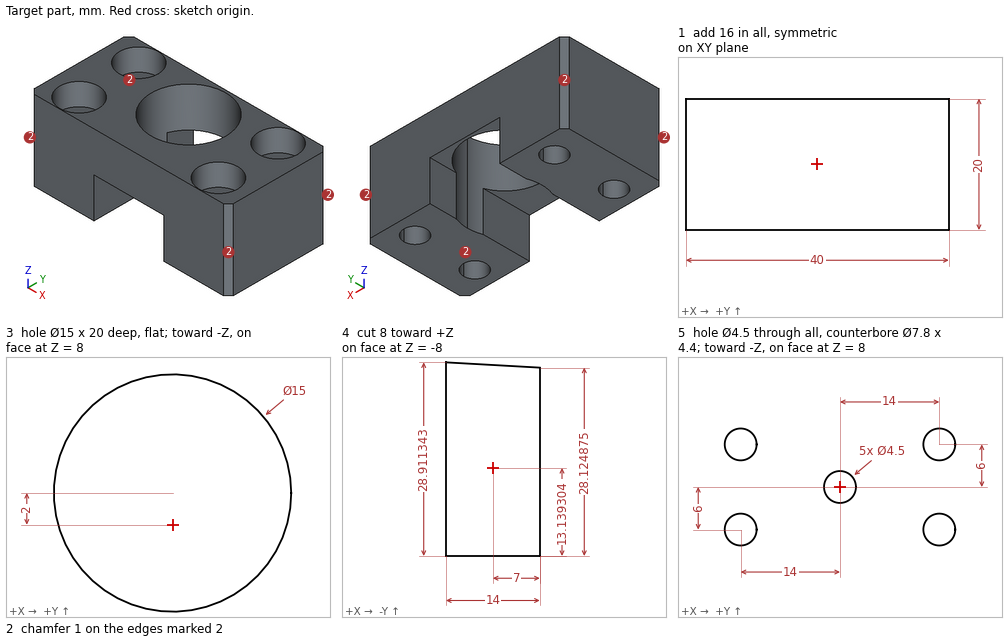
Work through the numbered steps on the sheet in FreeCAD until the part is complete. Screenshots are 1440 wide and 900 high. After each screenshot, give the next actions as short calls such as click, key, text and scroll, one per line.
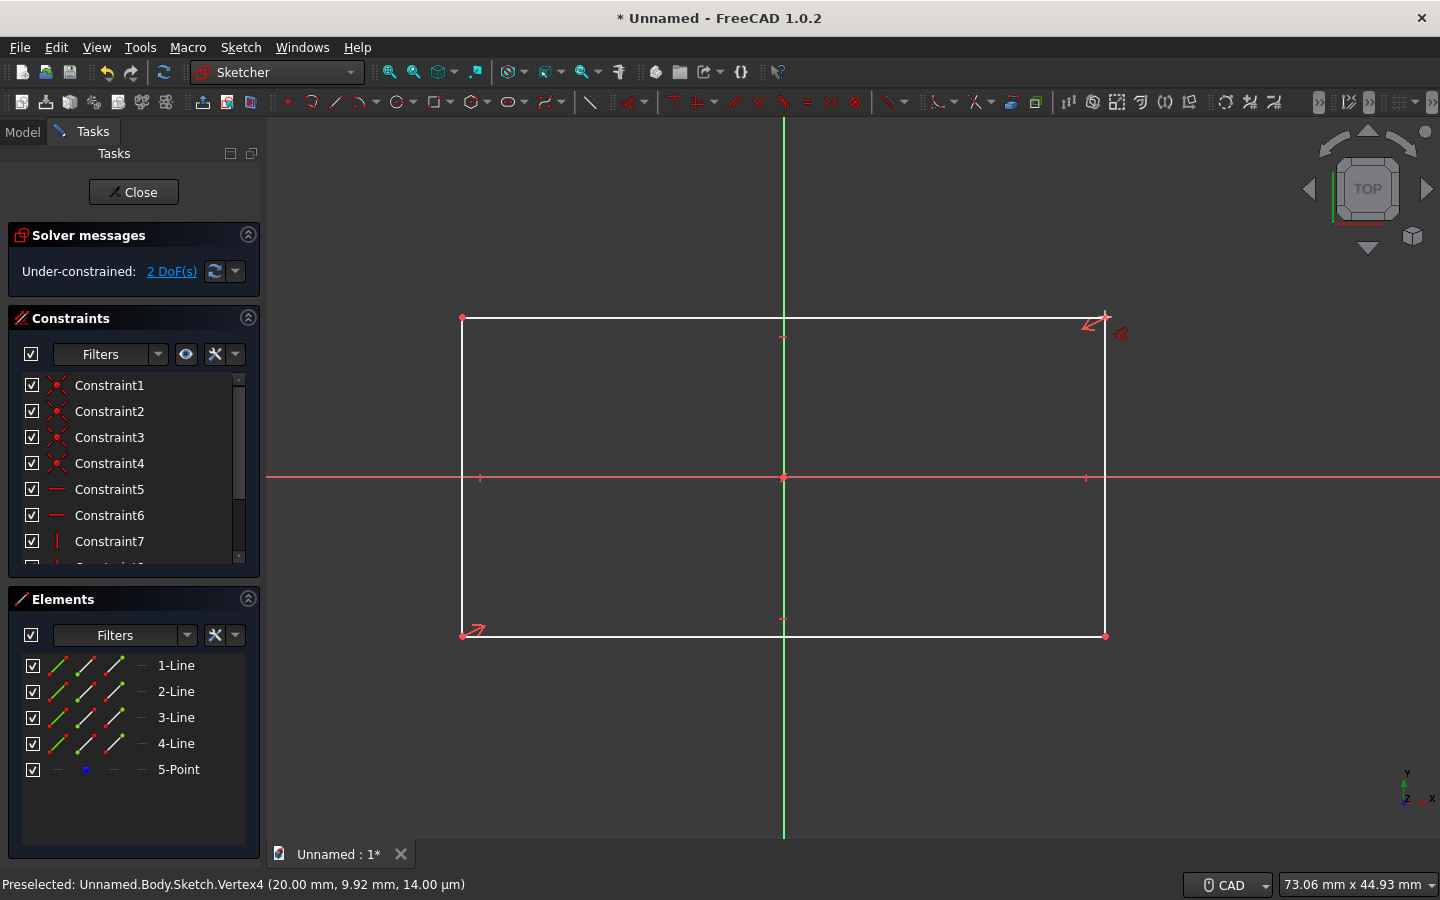
click(655, 637)
click(636, 671)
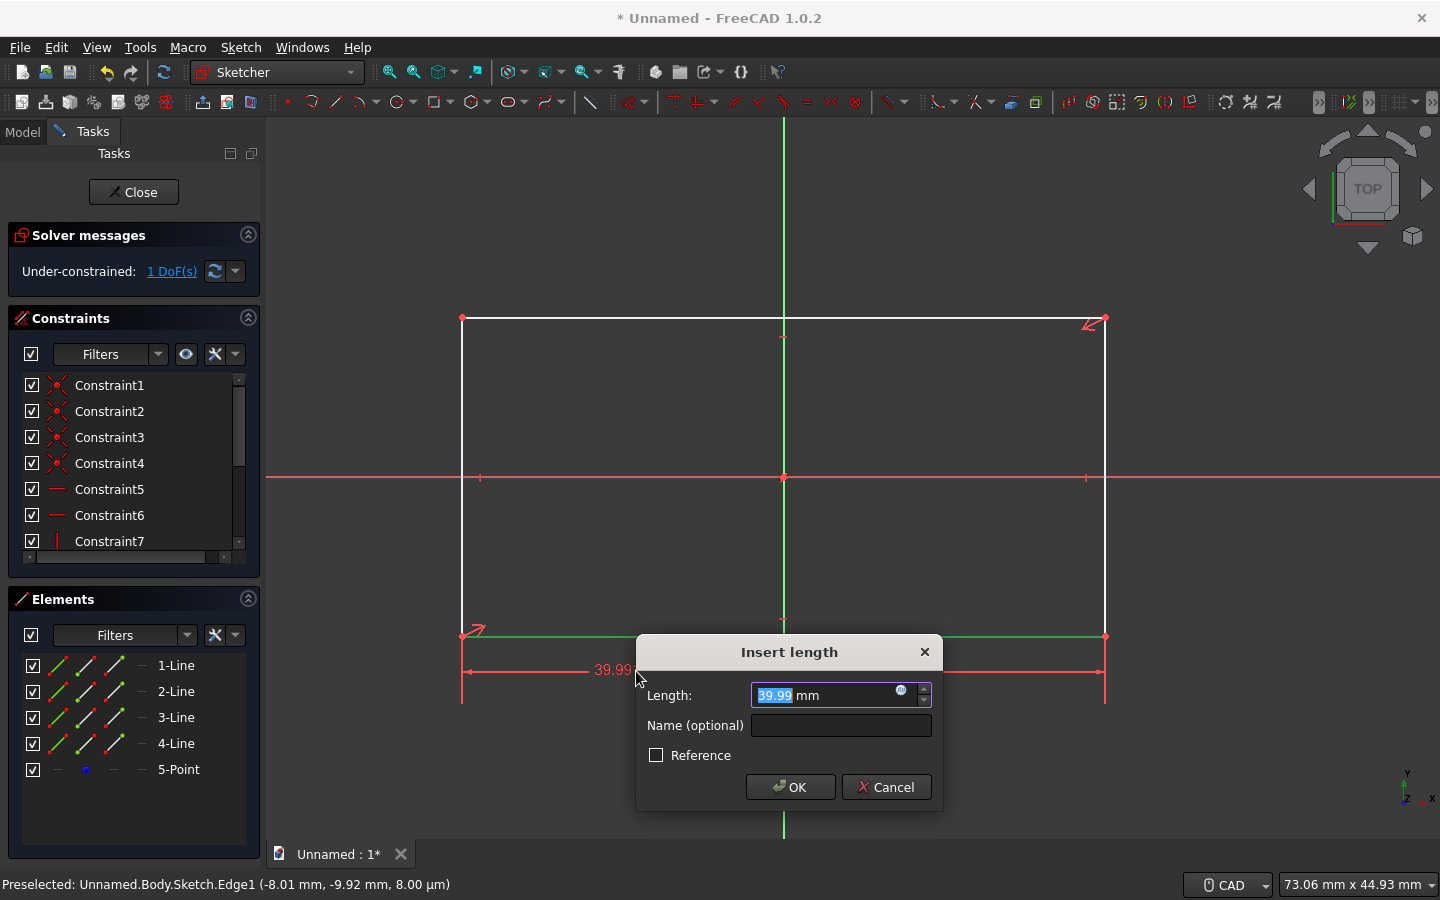
text(40)
key(Return)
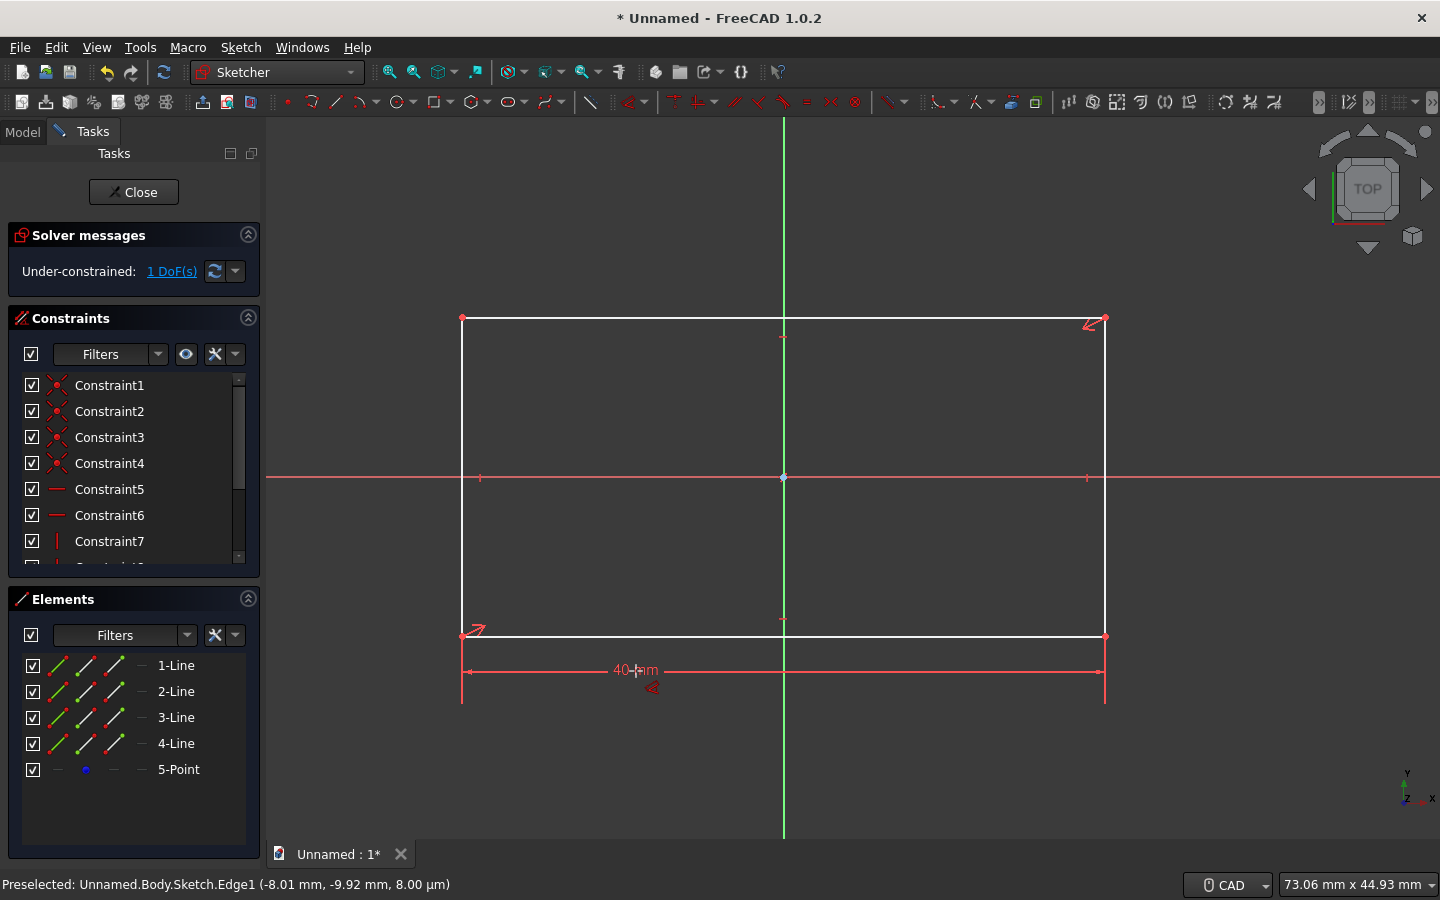
click(1105, 541)
click(1139, 404)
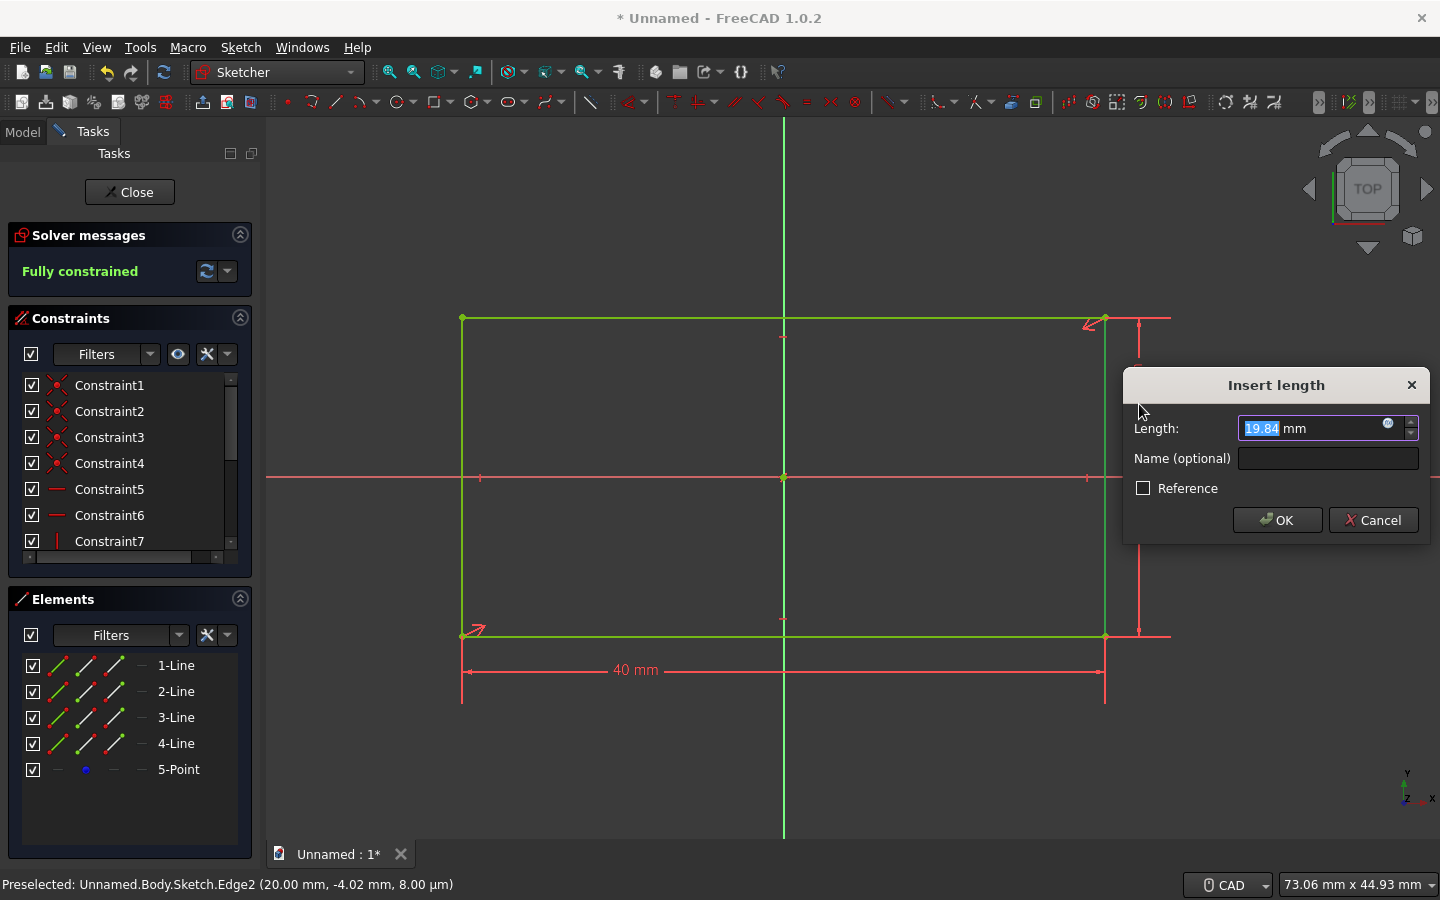
text(20)
key(Return)
key(Escape)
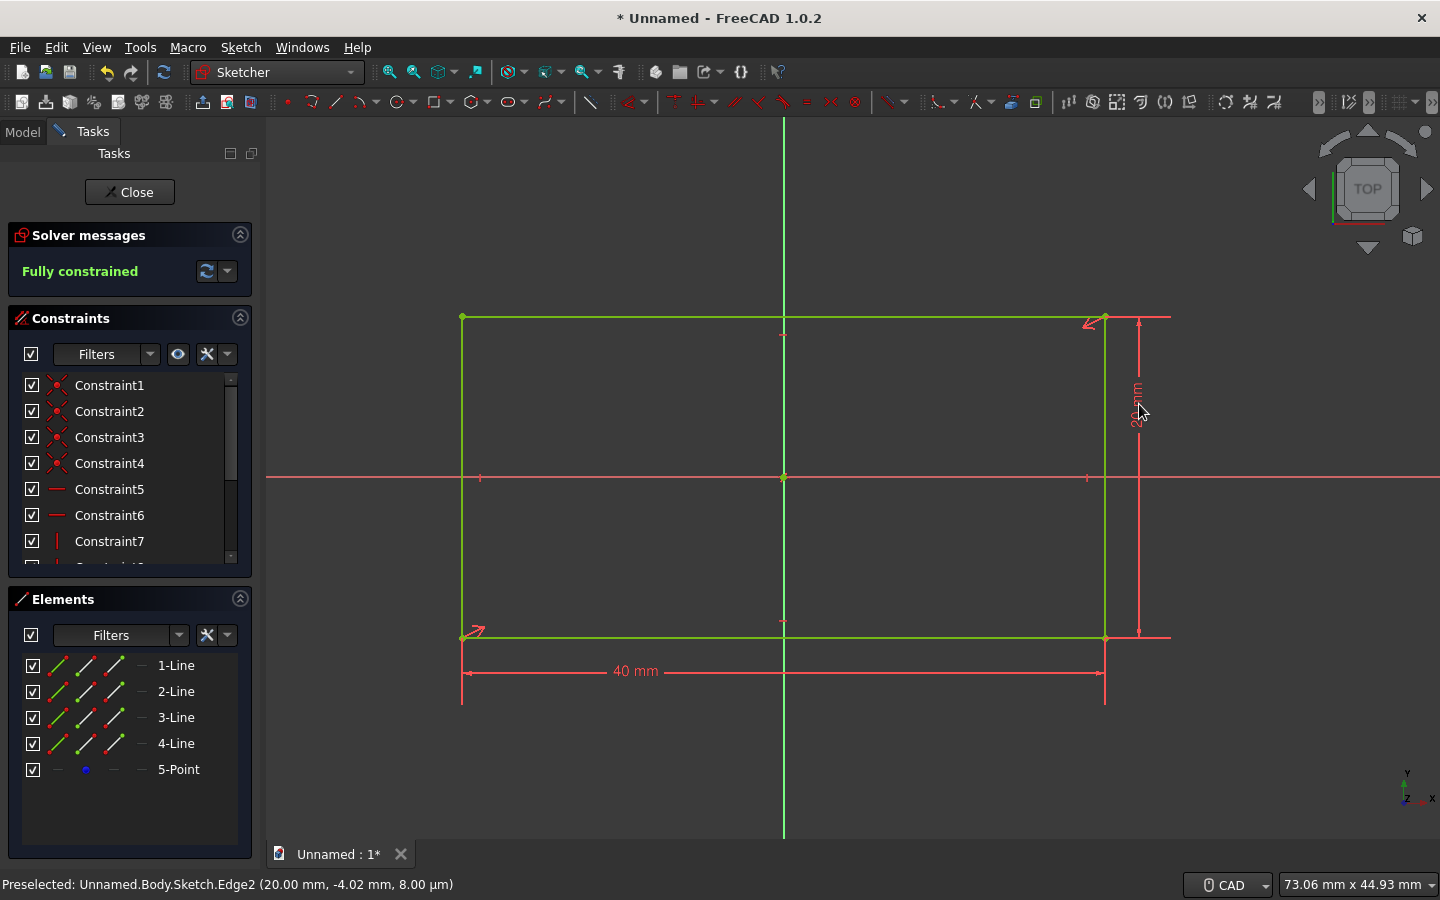
click(130, 192)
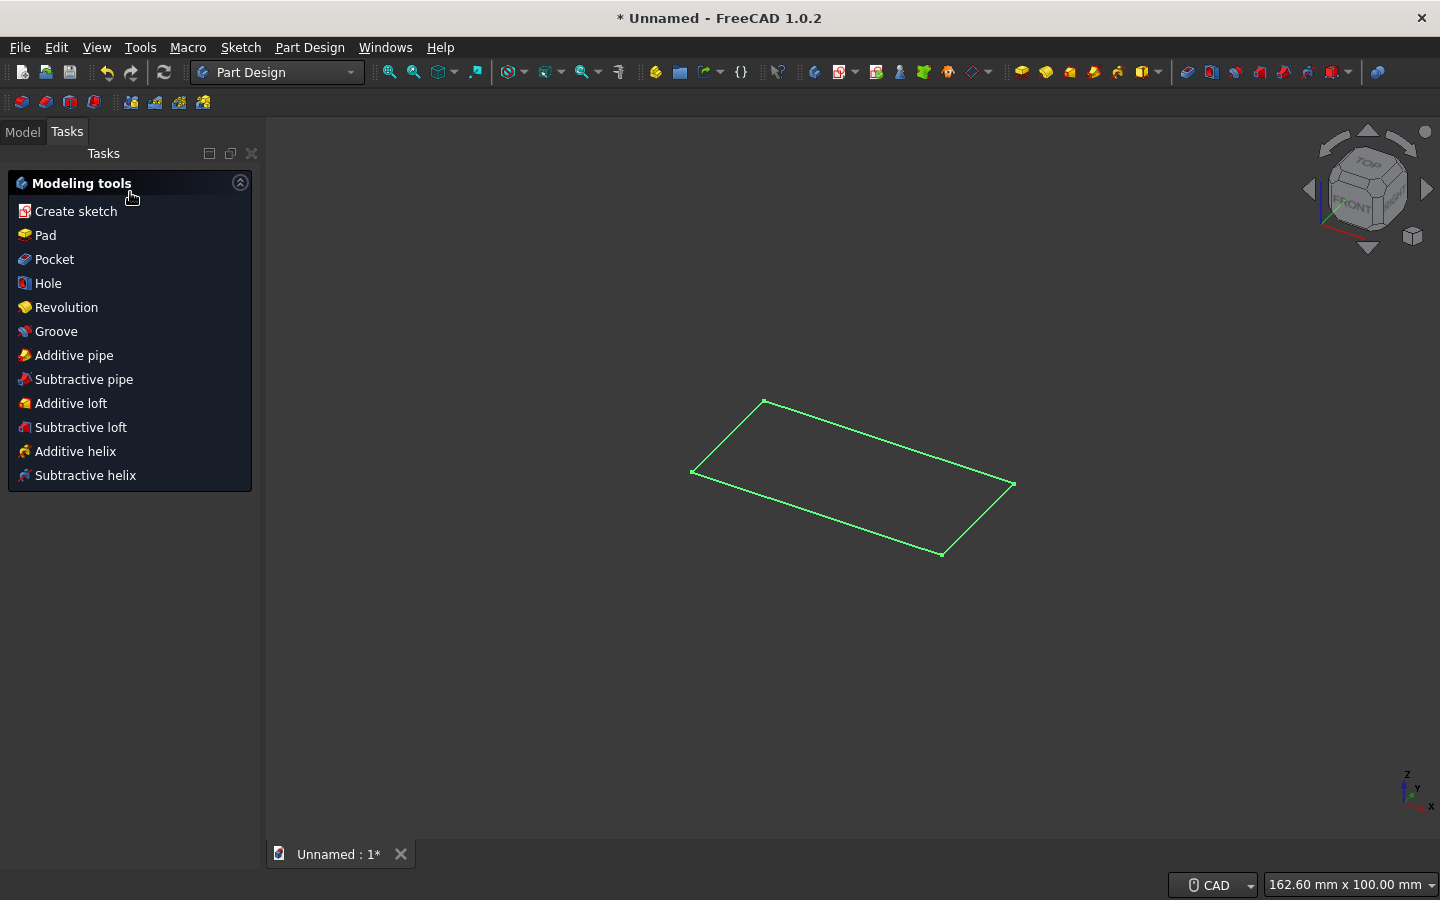
click(1022, 72)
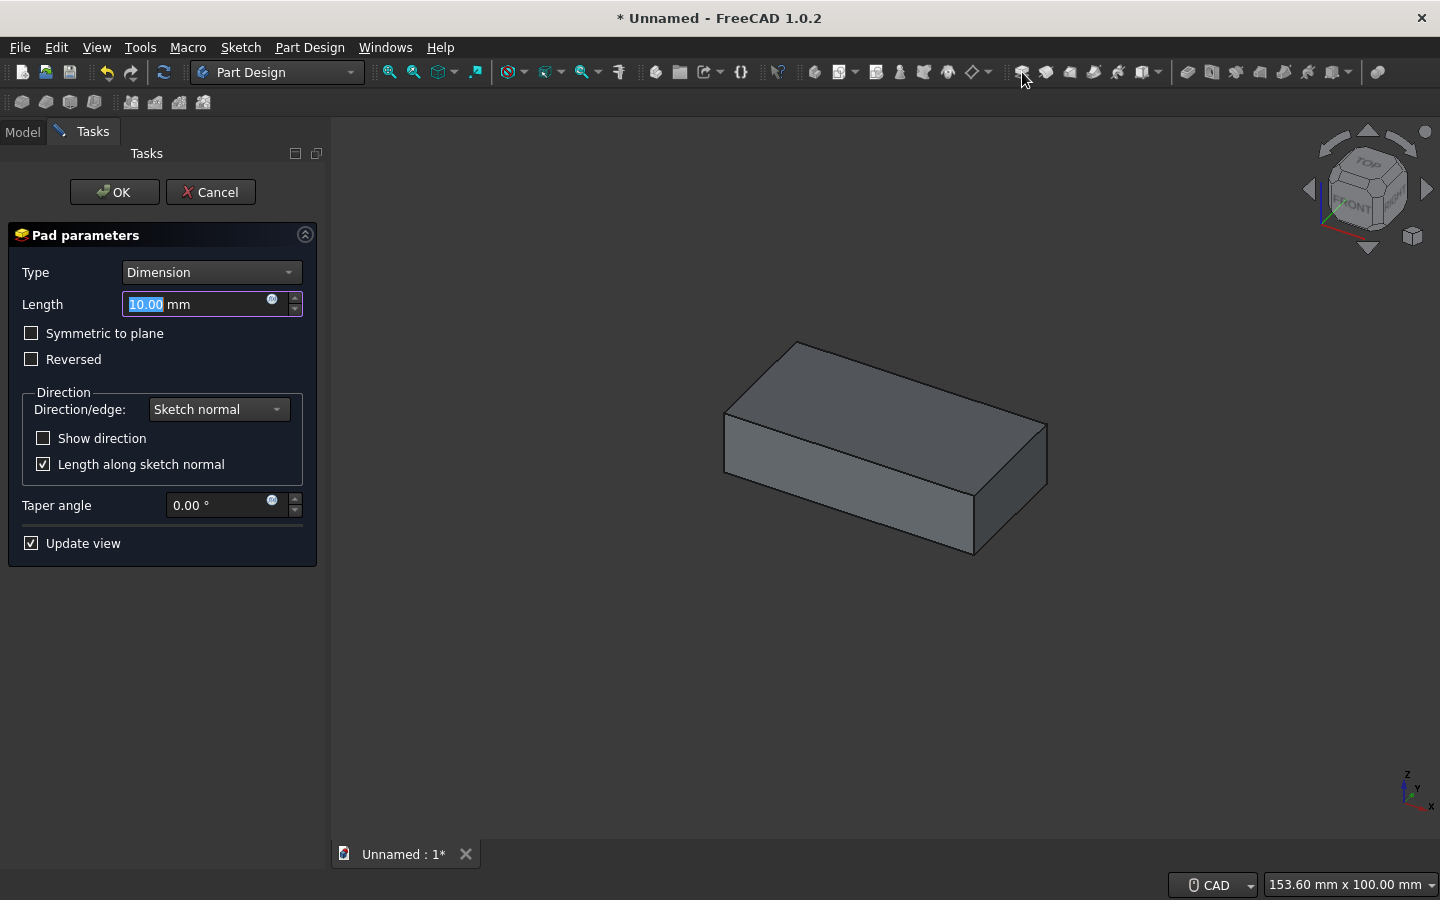
text(16)
key(Tab)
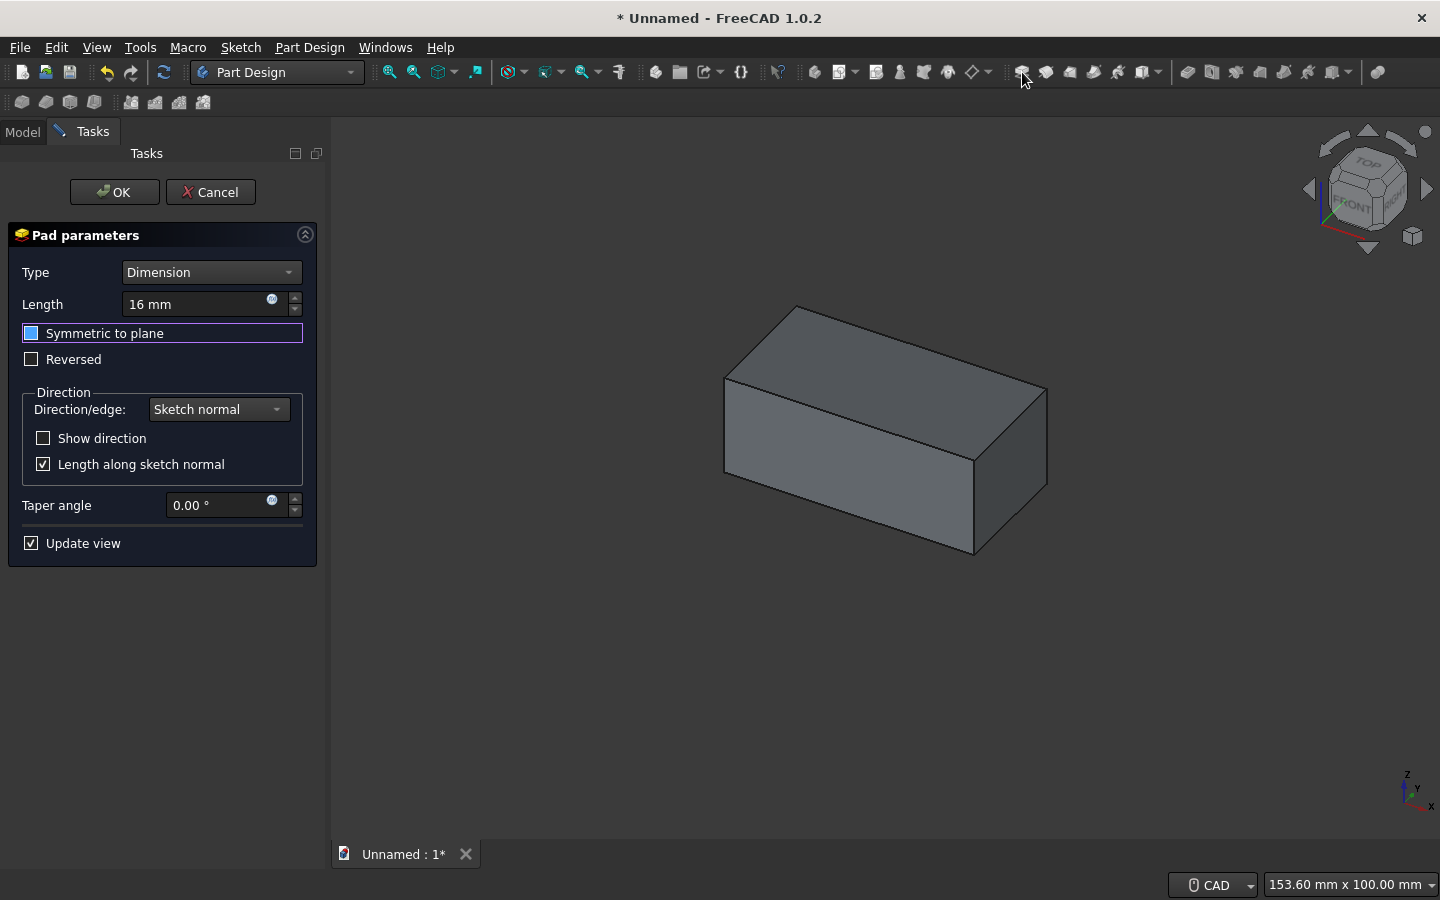
click(30, 333)